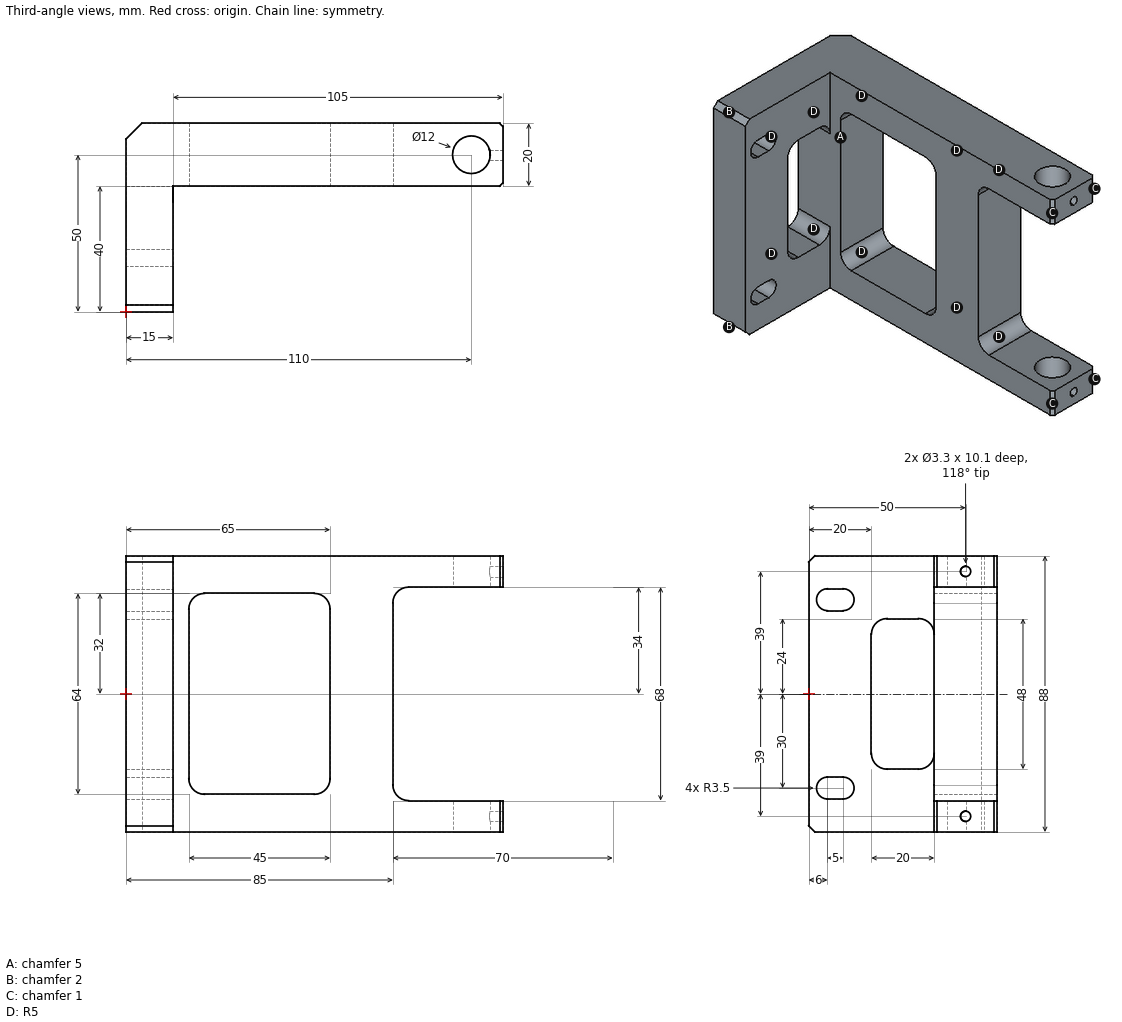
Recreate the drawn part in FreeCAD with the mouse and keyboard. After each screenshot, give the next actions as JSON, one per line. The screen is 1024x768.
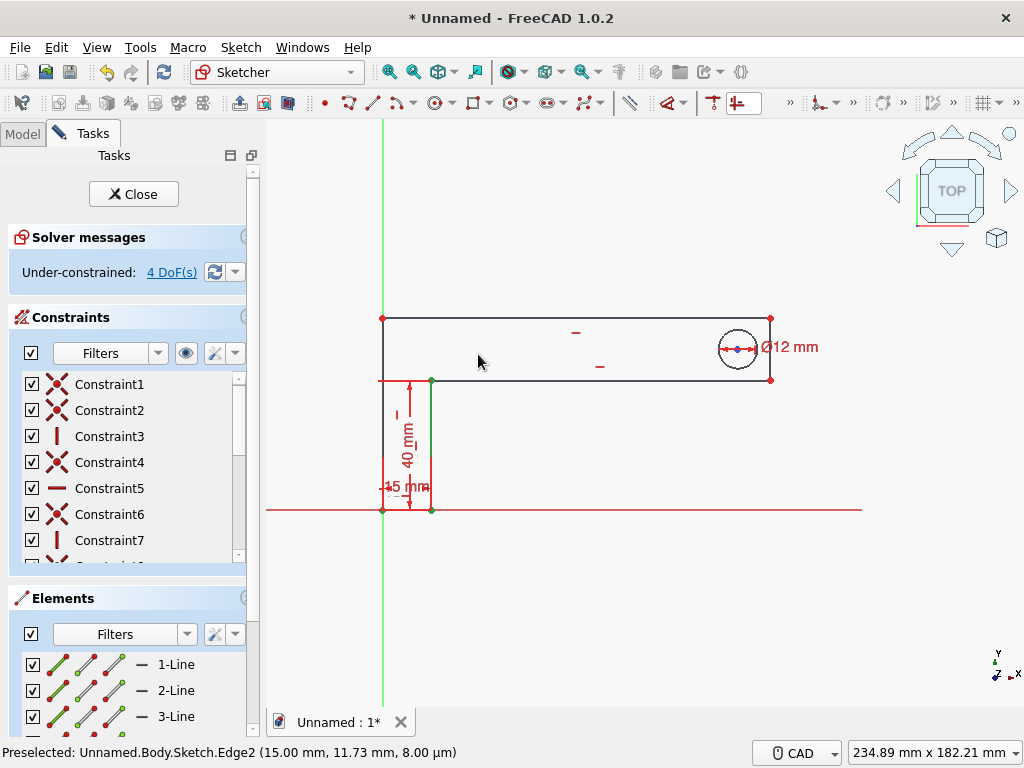
{"action": "left_click", "coordinate": [770, 362]}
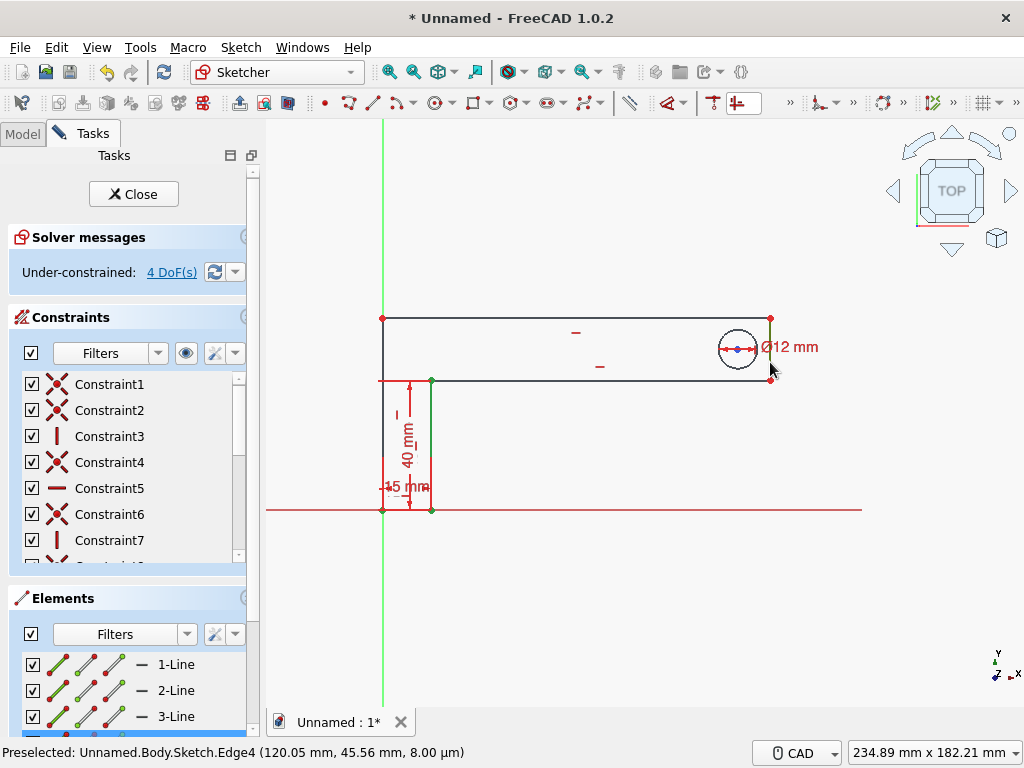
{"action": "left_click", "coordinate": [686, 104]}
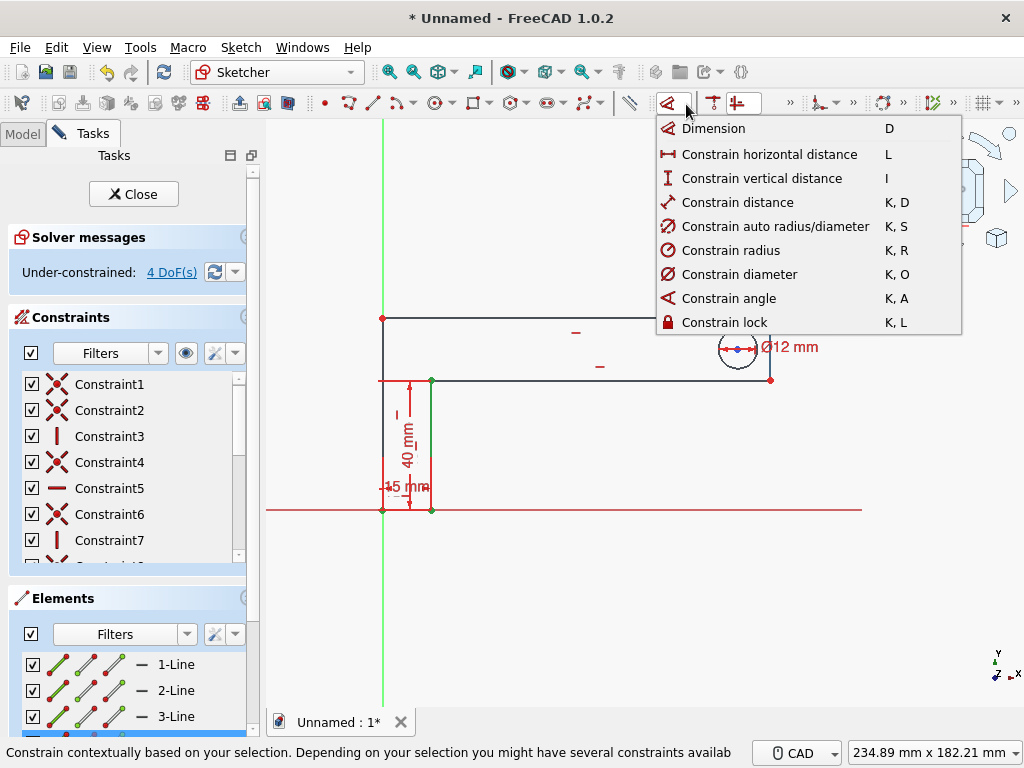
{"action": "left_click", "coordinate": [809, 178]}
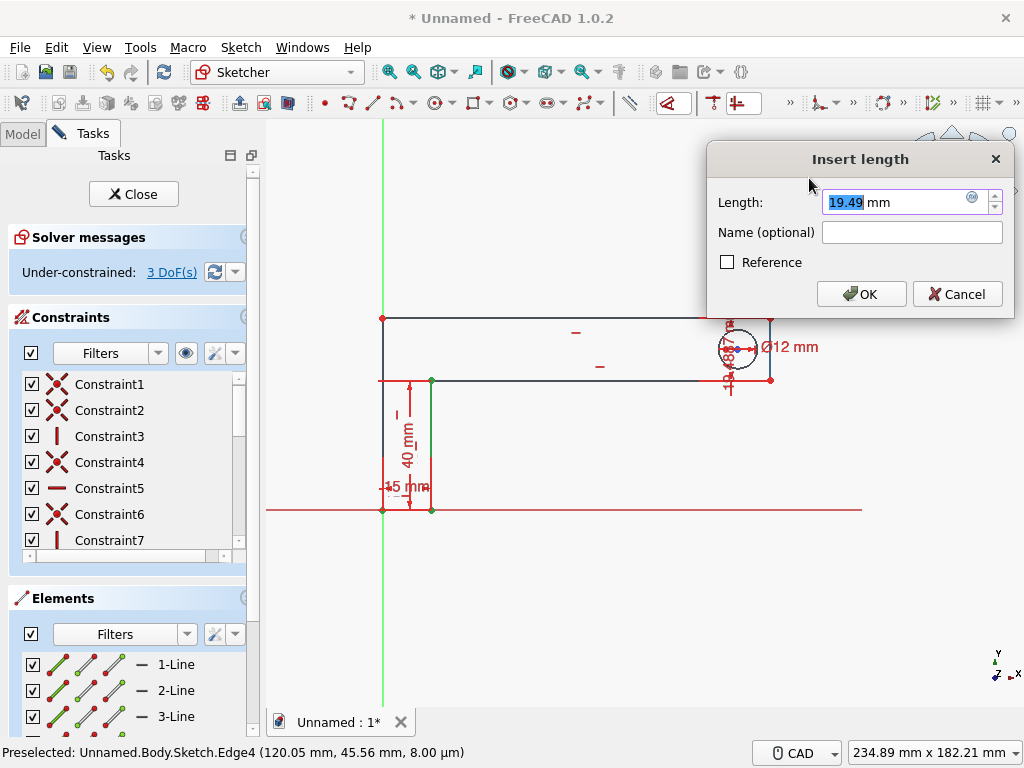
{"action": "type", "text": "20"}
{"action": "key", "text": "Return"}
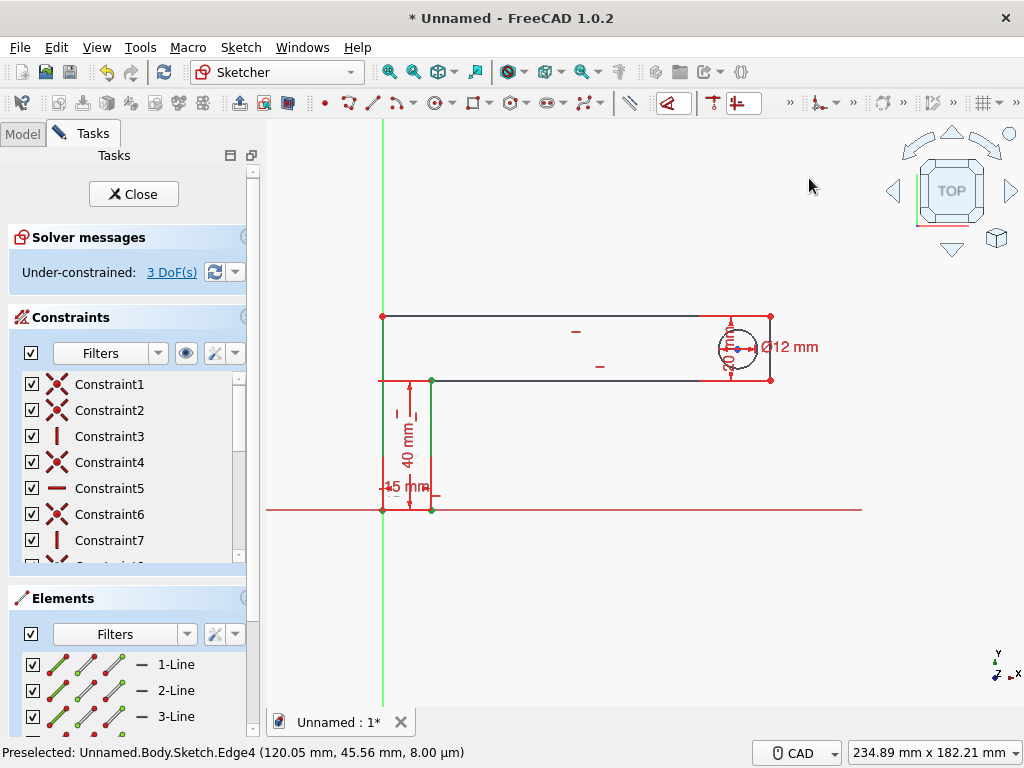
{"action": "left_click", "coordinate": [738, 349]}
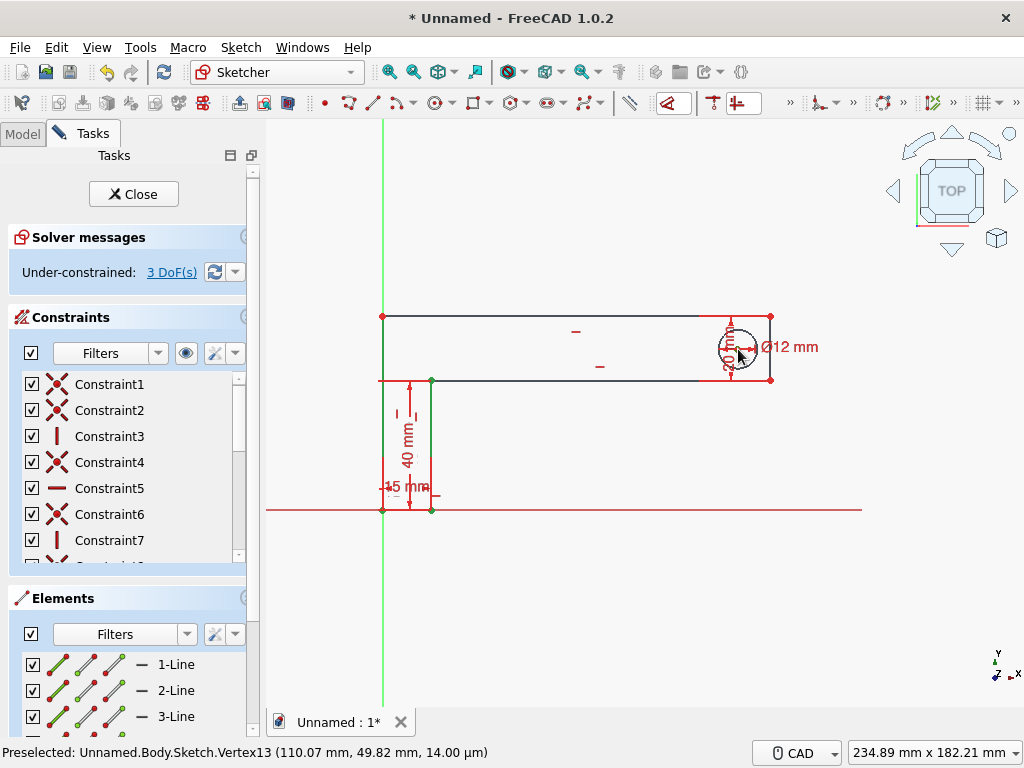
{"action": "key", "text": "i"}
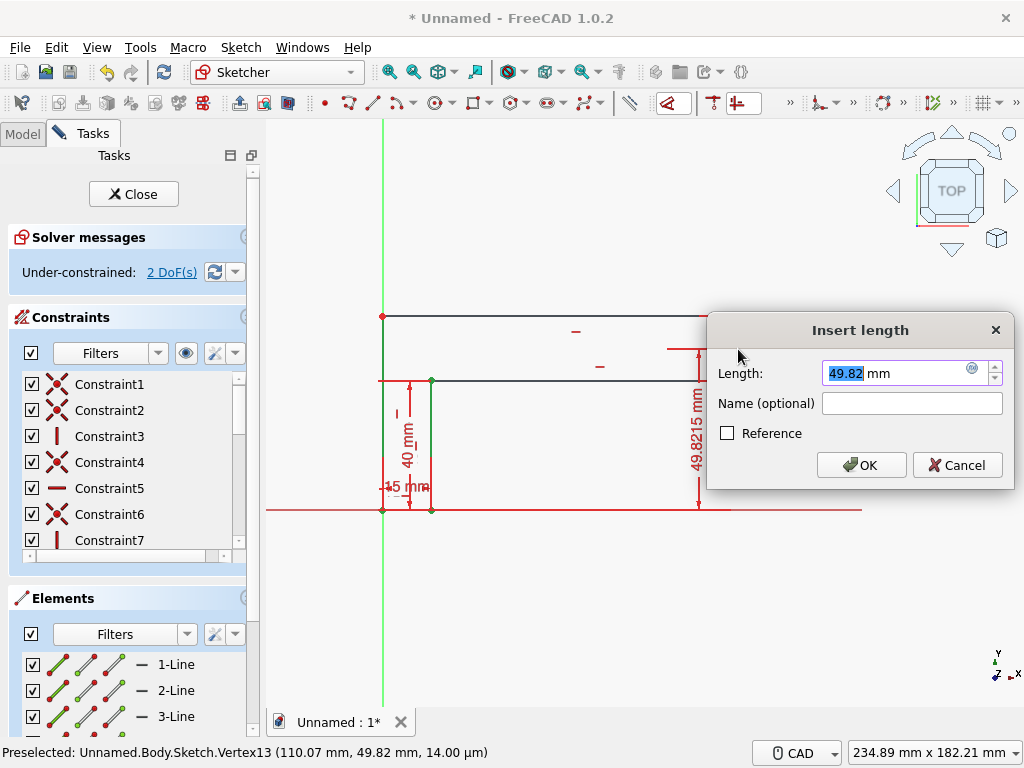
{"action": "type", "text": "50"}
{"action": "key", "text": "Return"}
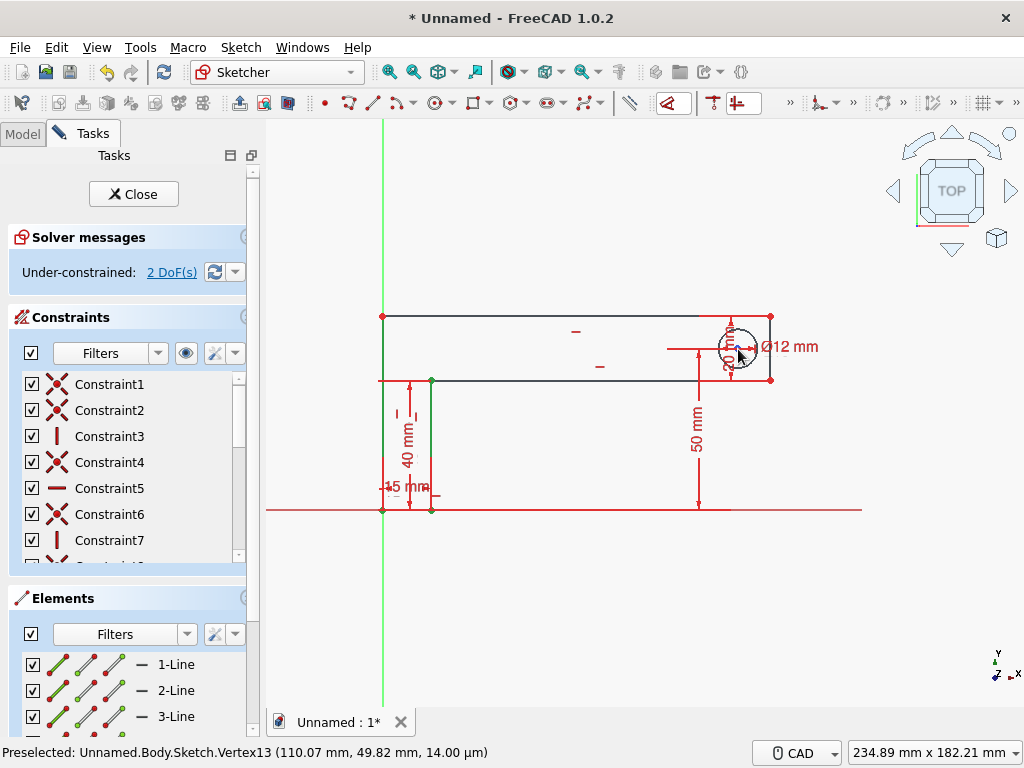
{"action": "left_click", "coordinate": [533, 381]}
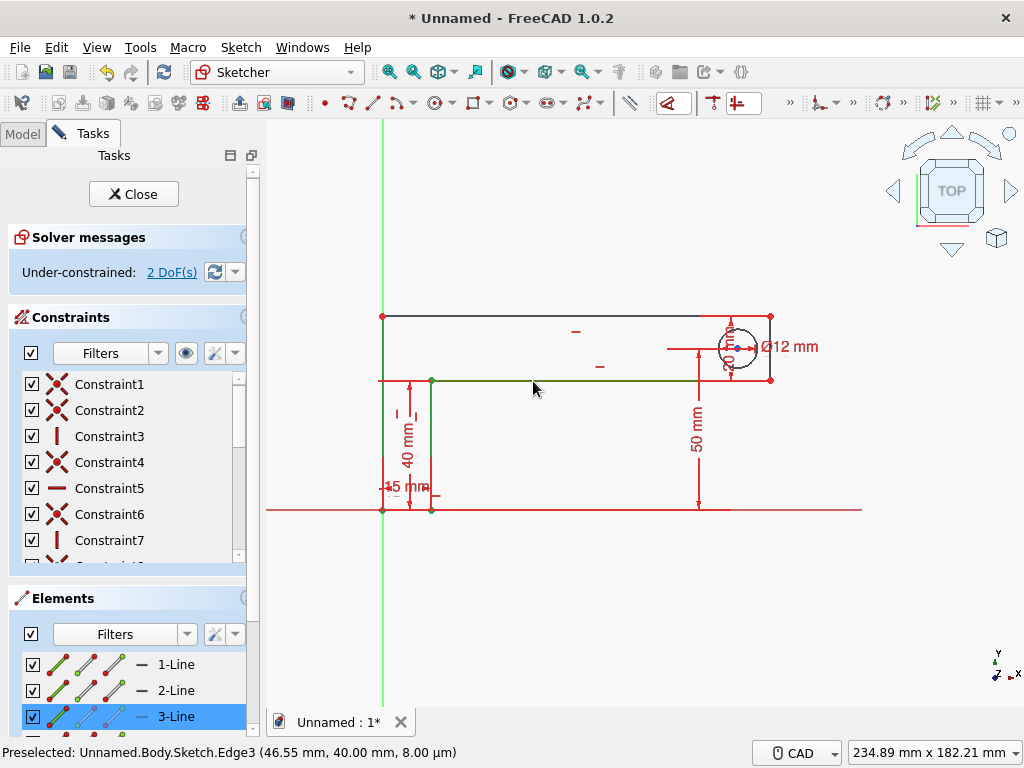
{"action": "key", "text": "l"}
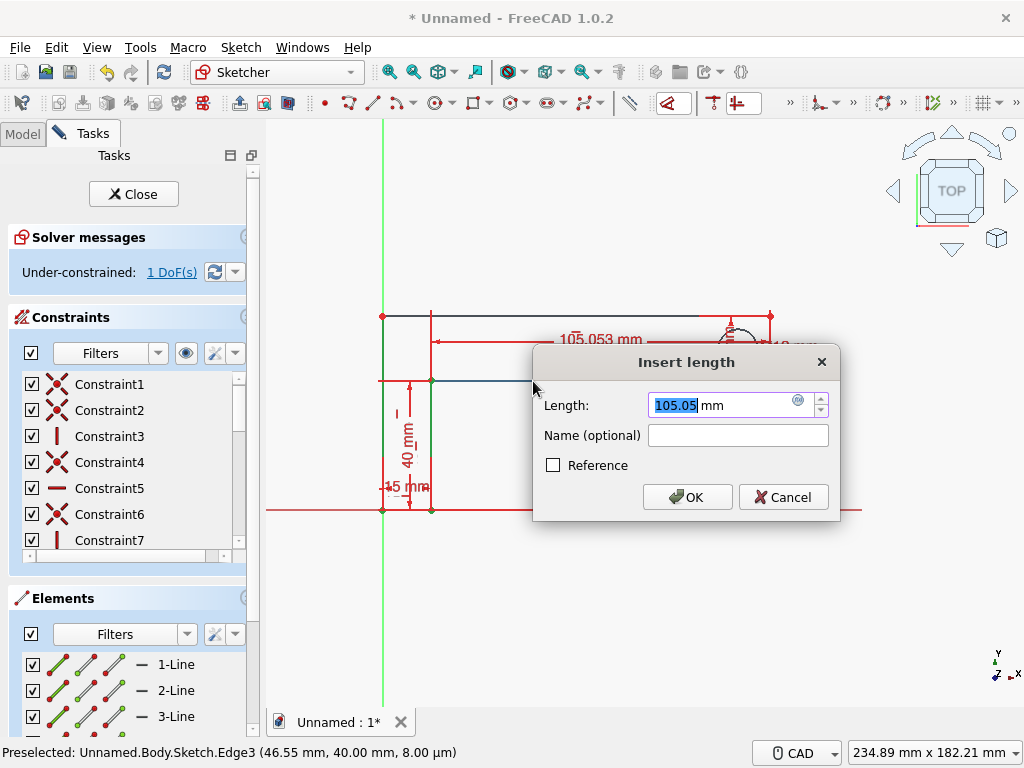
{"action": "type", "text": "105"}
{"action": "key", "text": "Return"}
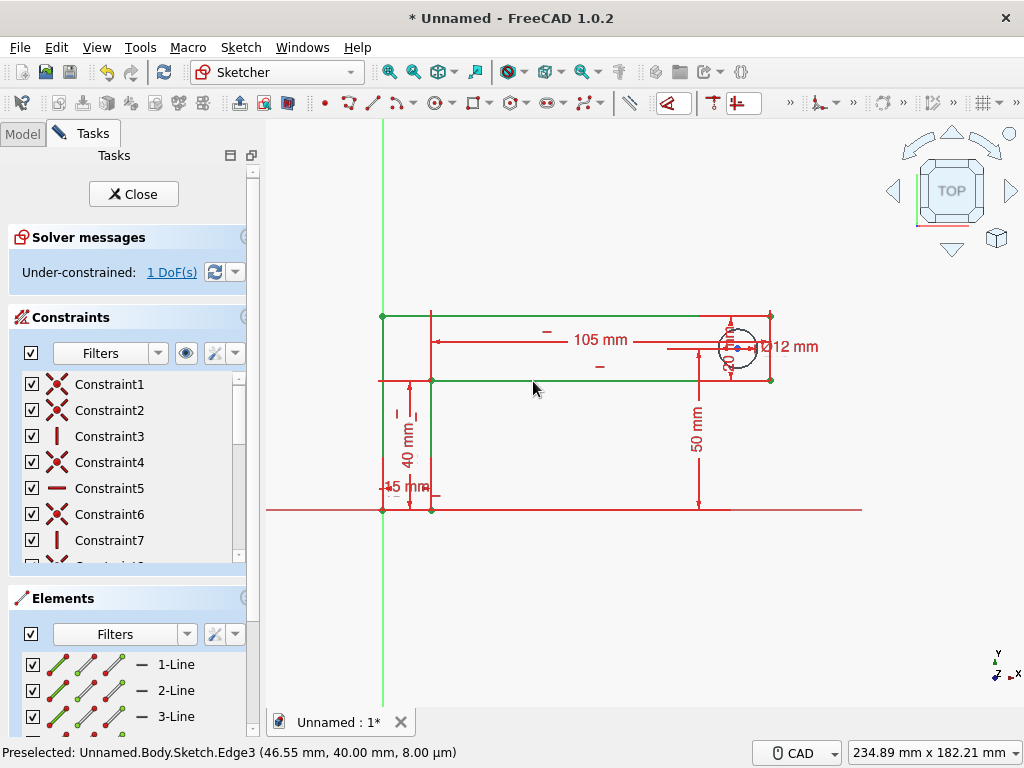
{"action": "left_click", "coordinate": [738, 349]}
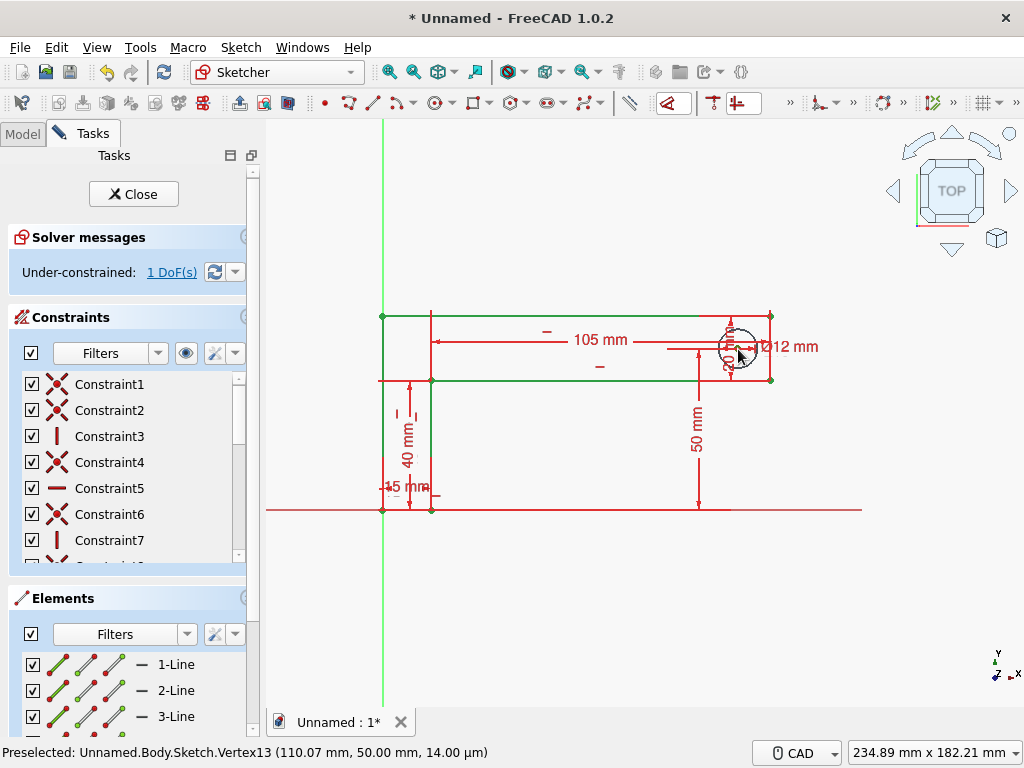
{"action": "key", "text": "l"}